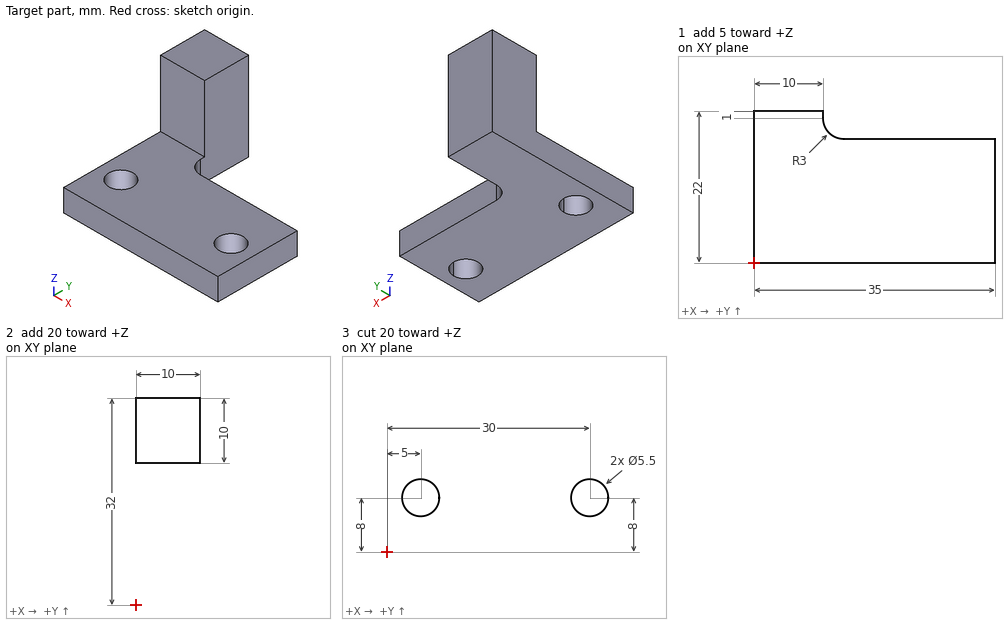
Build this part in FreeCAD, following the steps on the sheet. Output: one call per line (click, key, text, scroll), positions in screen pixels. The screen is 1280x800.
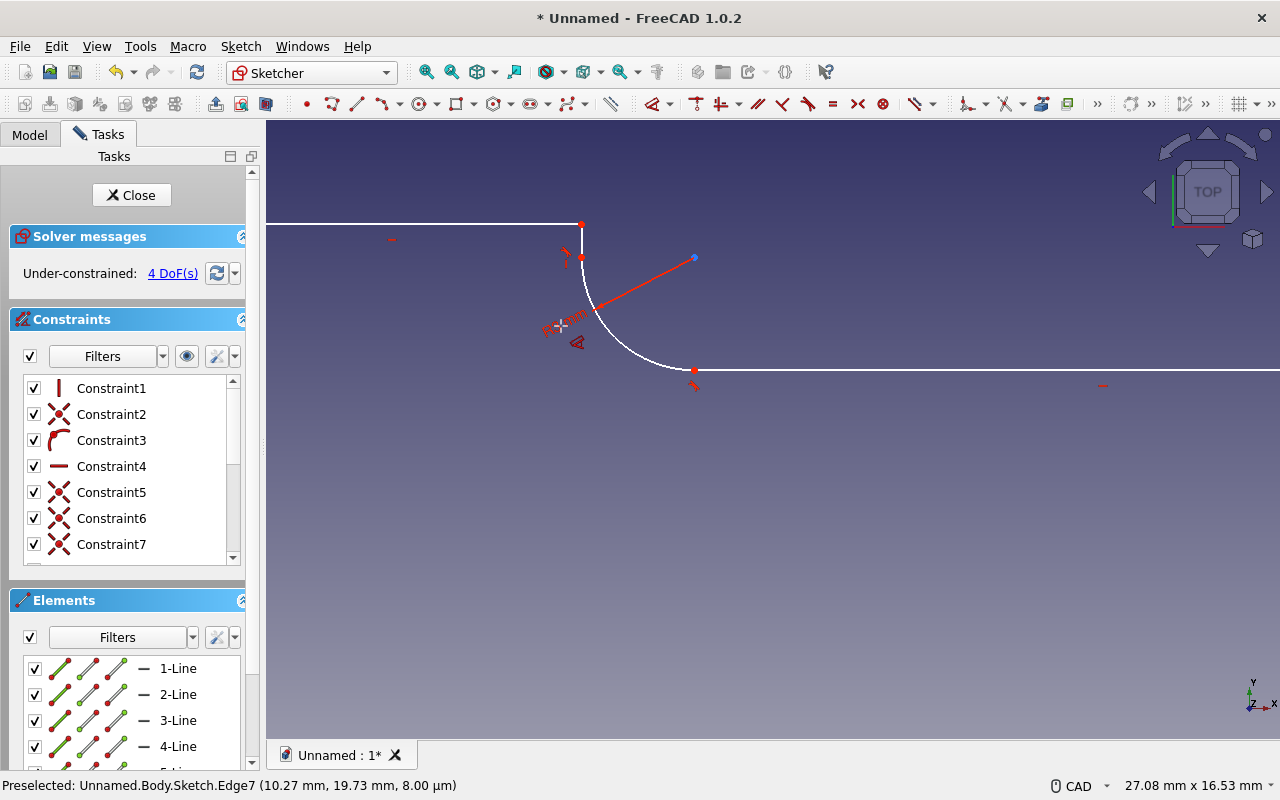
scroll(582, 248, up, 2)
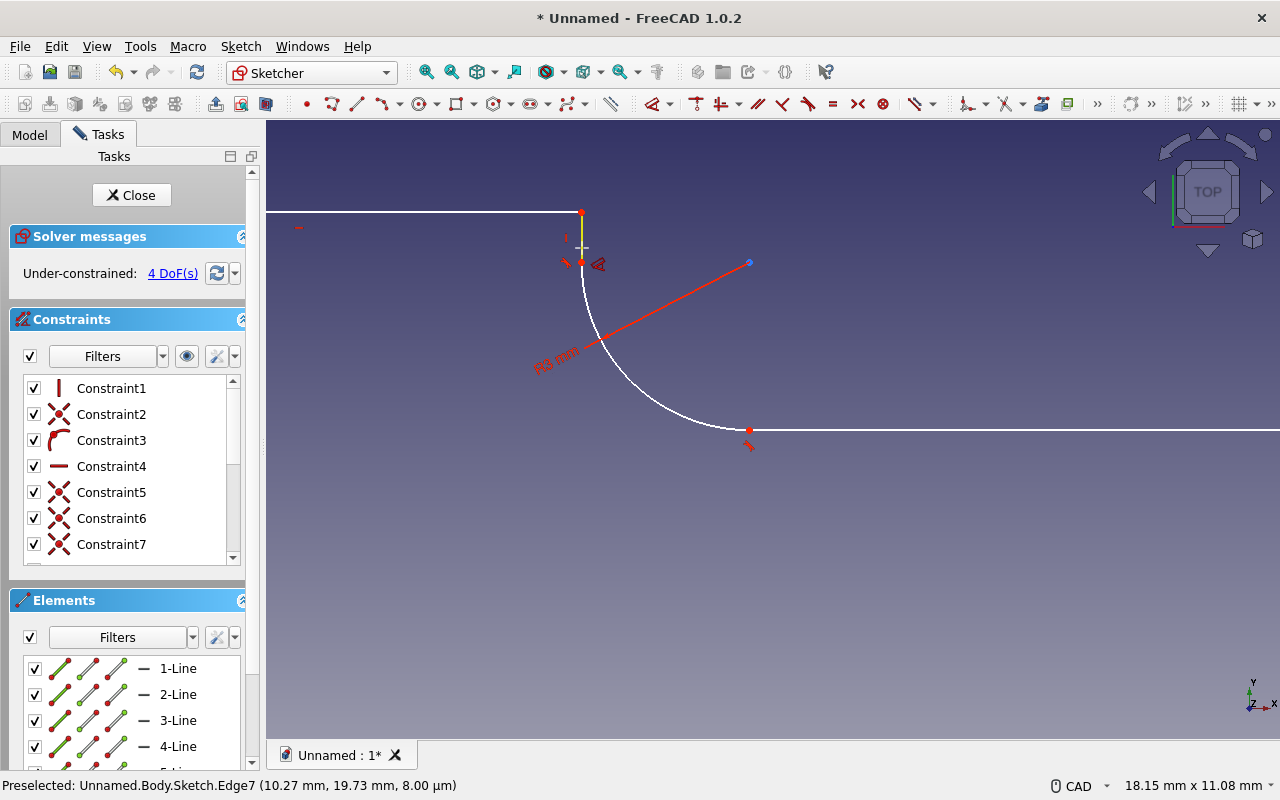
click(582, 247)
click(548, 237)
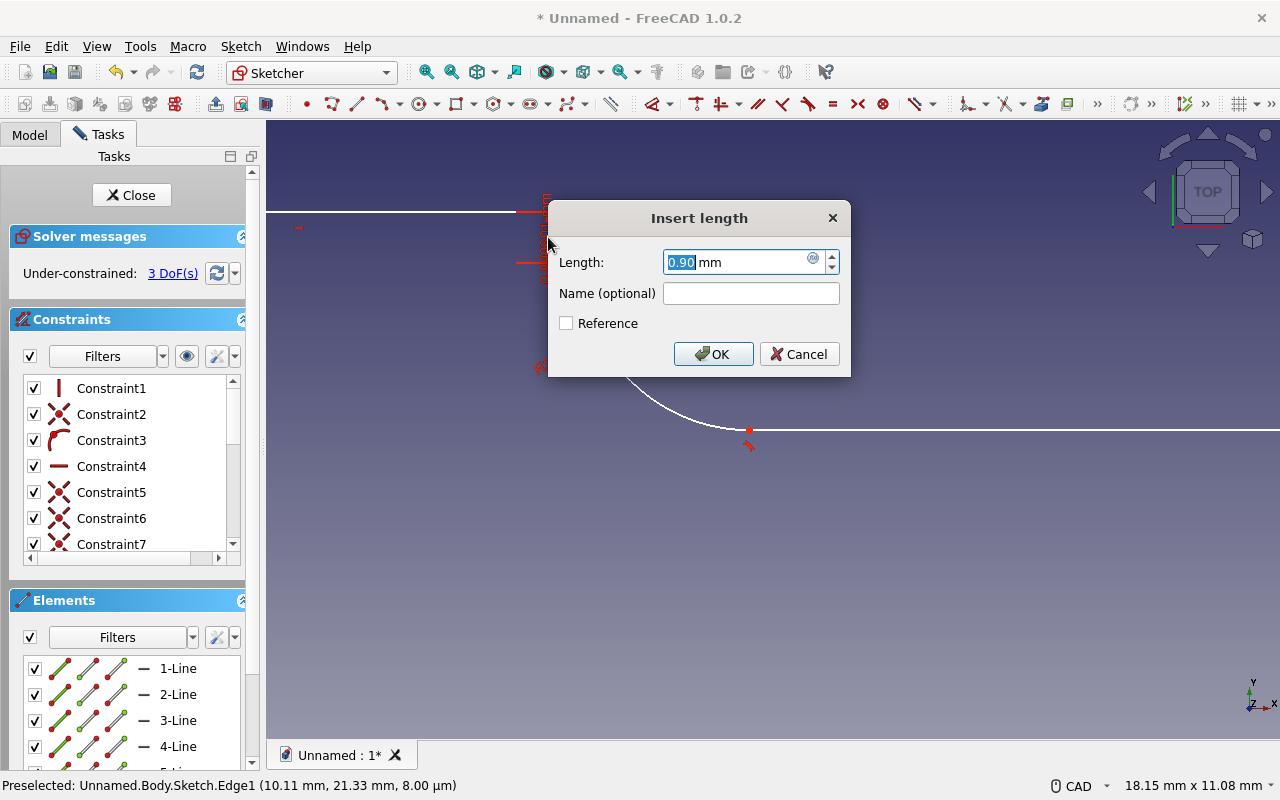
text(1)
key(Return)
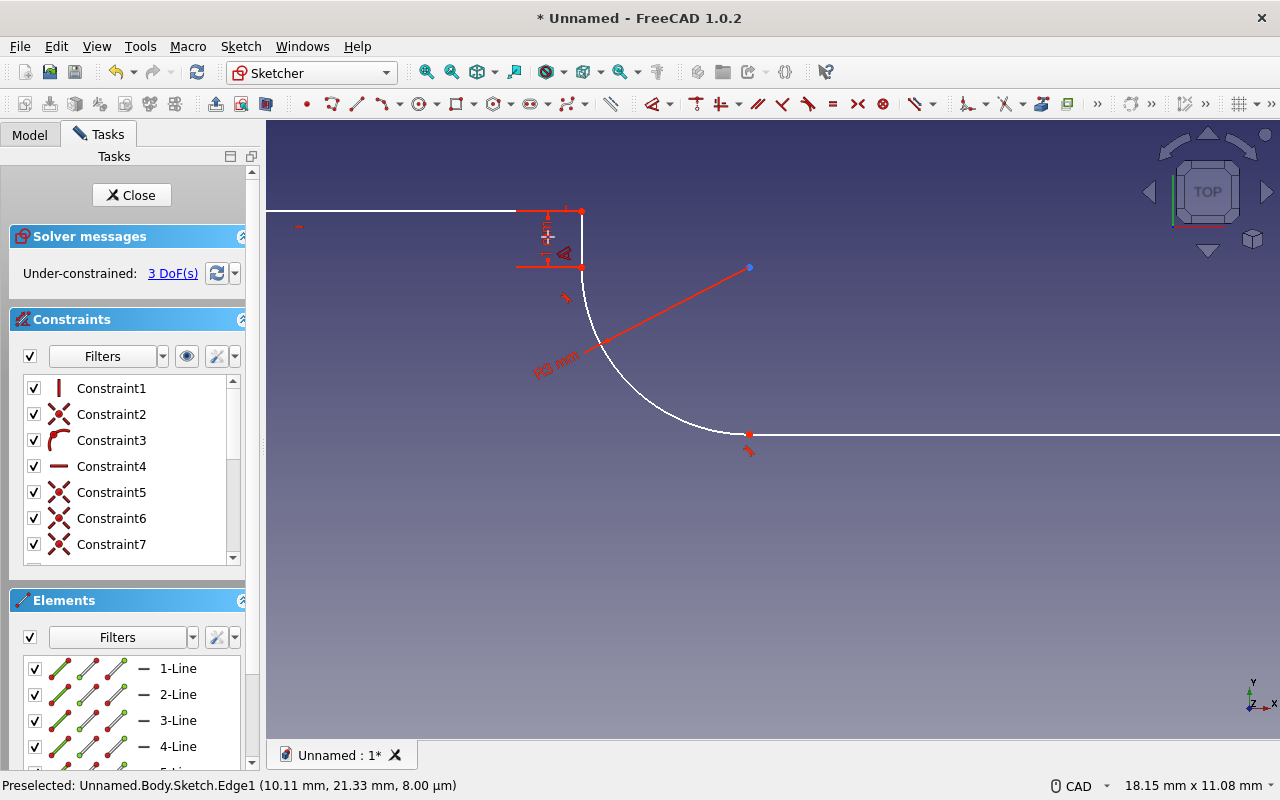
click(412, 211)
click(438, 177)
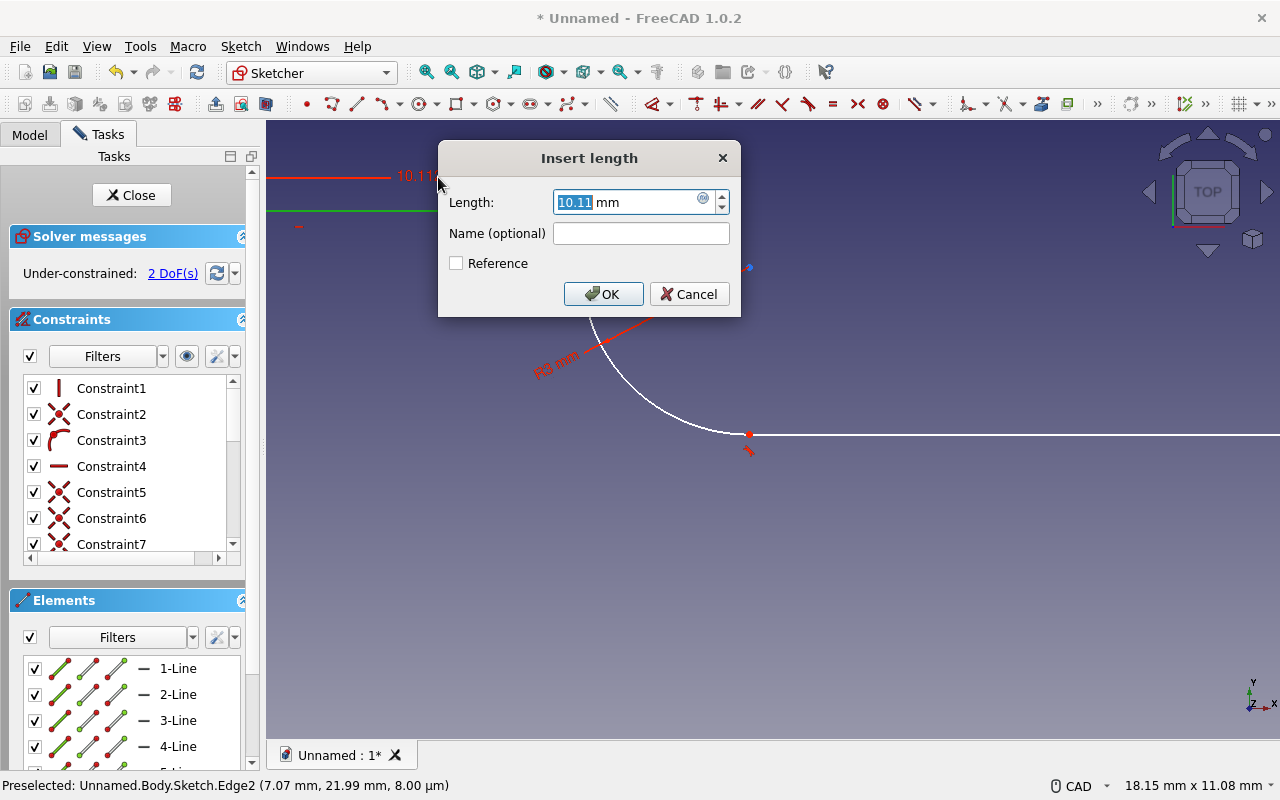
text(10)
key(Return)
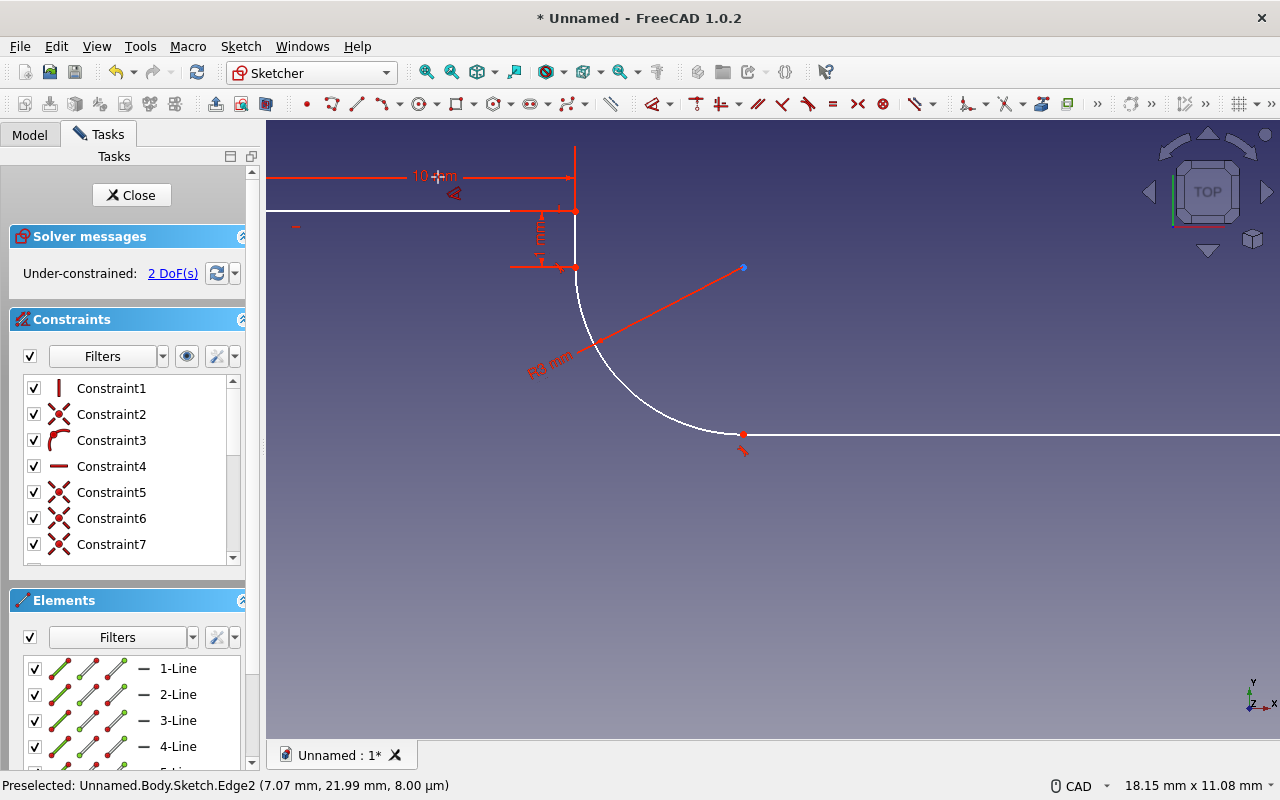
scroll(580, 259, down, 6)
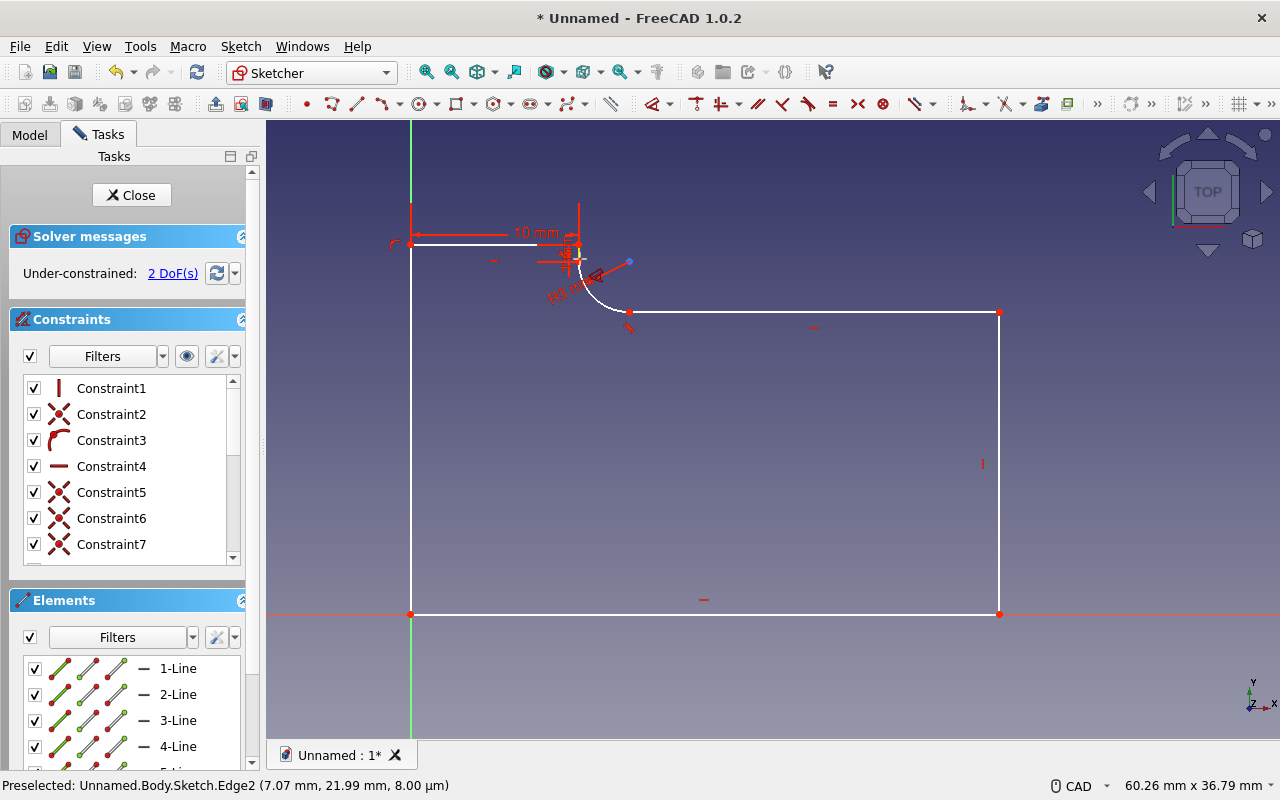
click(411, 356)
click(377, 430)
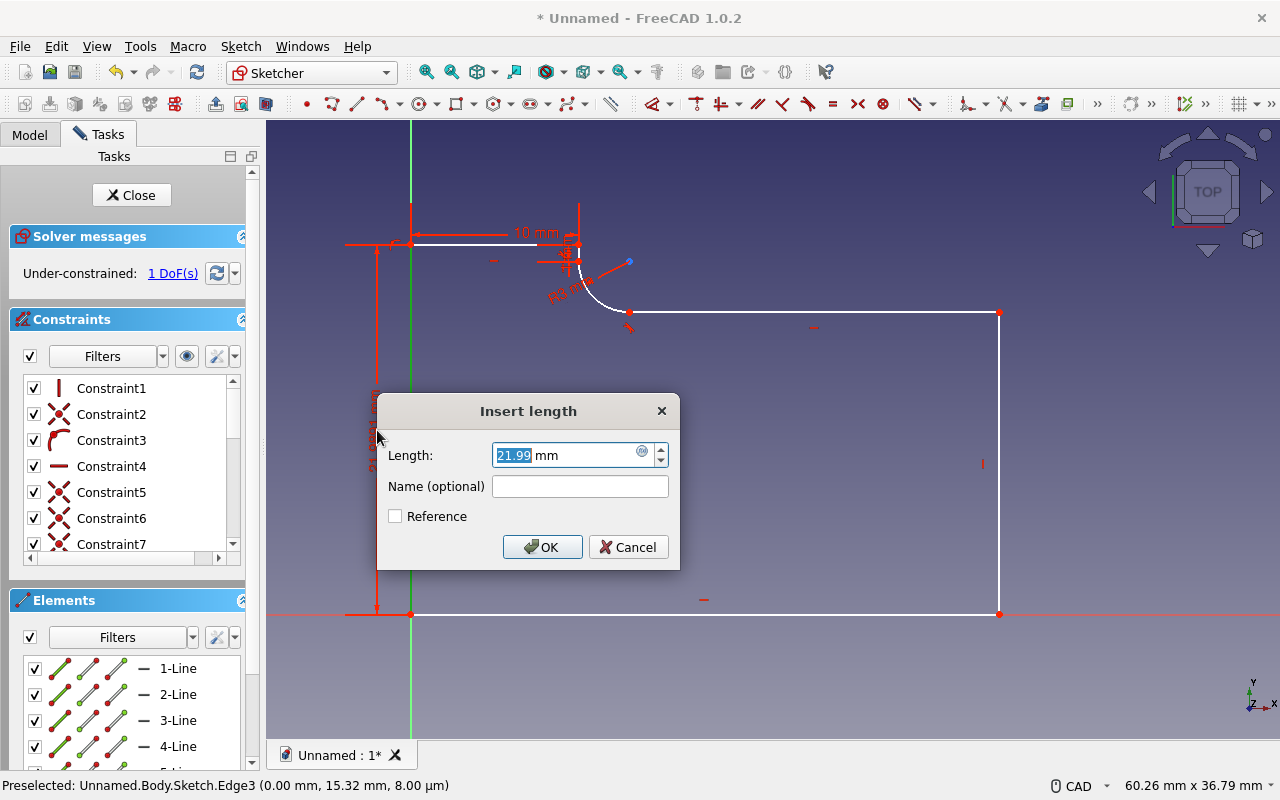
text(22)
key(Return)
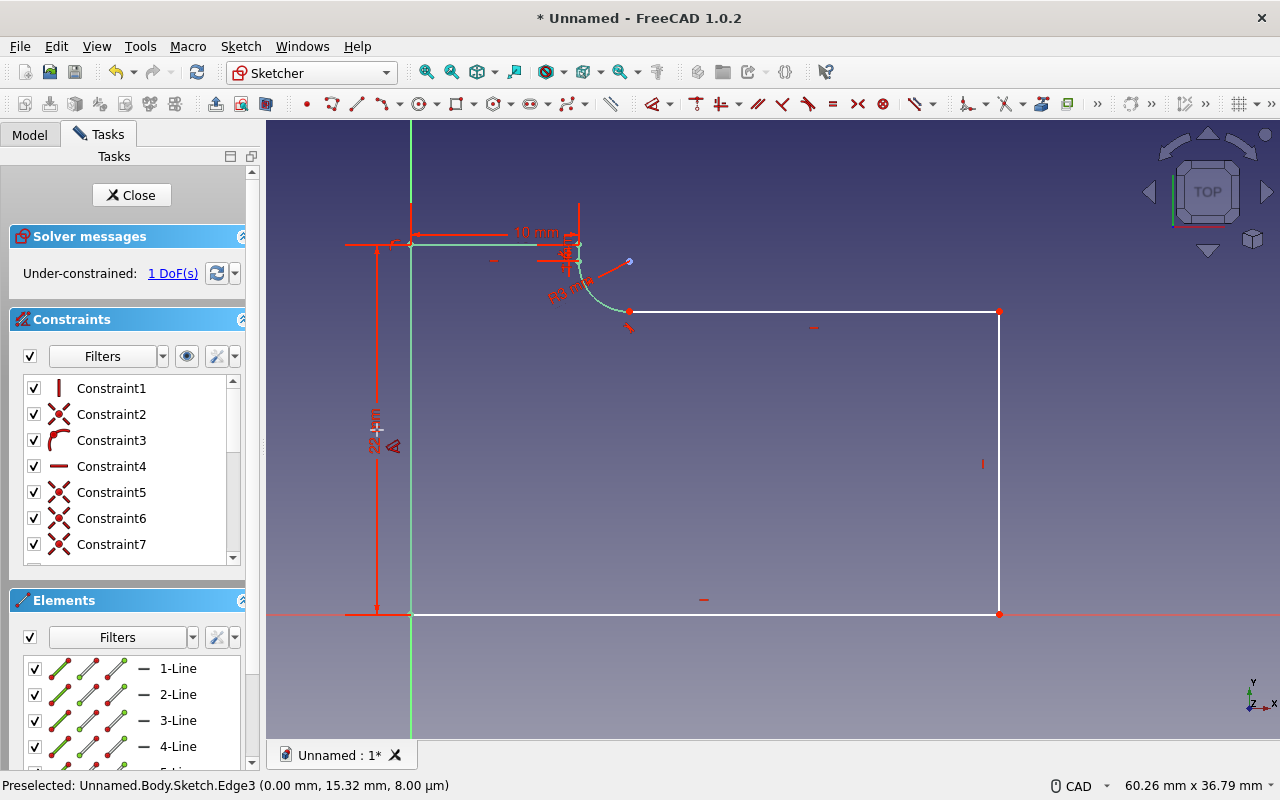
click(587, 615)
click(705, 649)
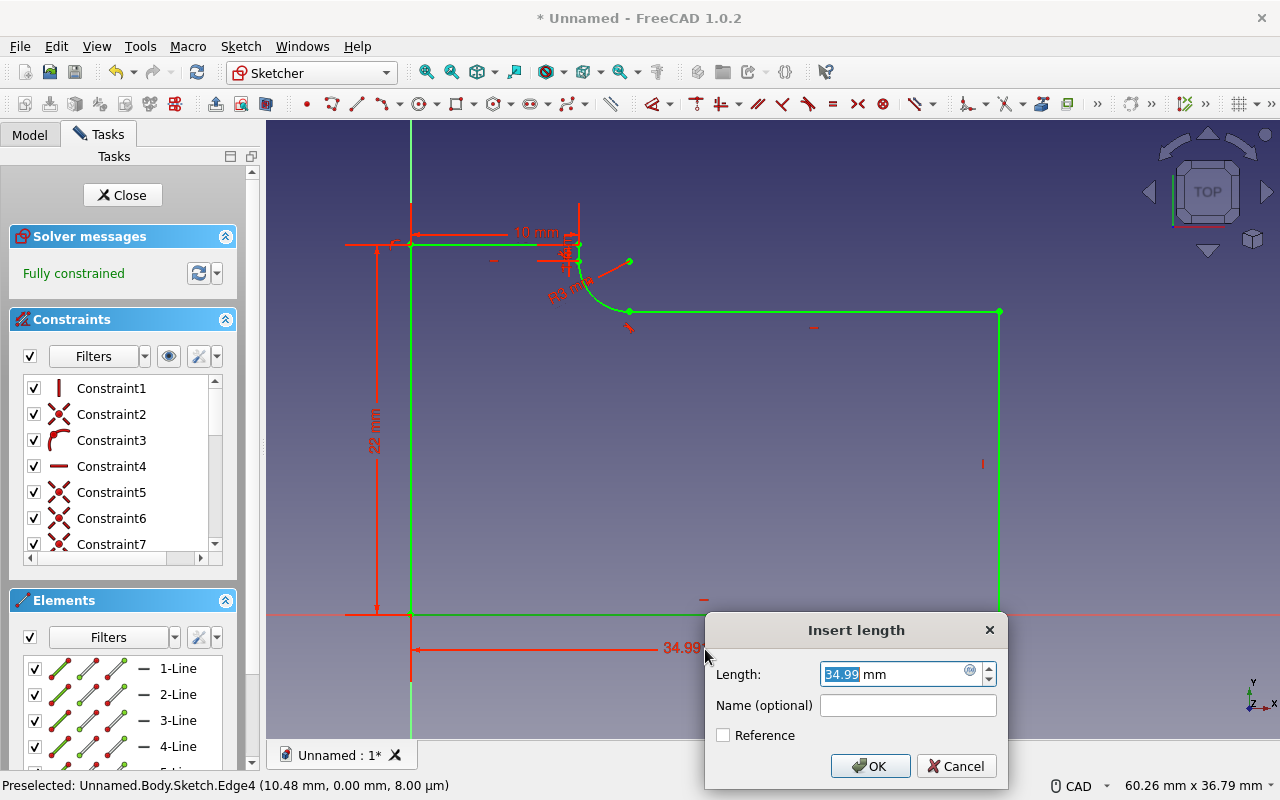
text(35)
key(Return)
key(Escape)